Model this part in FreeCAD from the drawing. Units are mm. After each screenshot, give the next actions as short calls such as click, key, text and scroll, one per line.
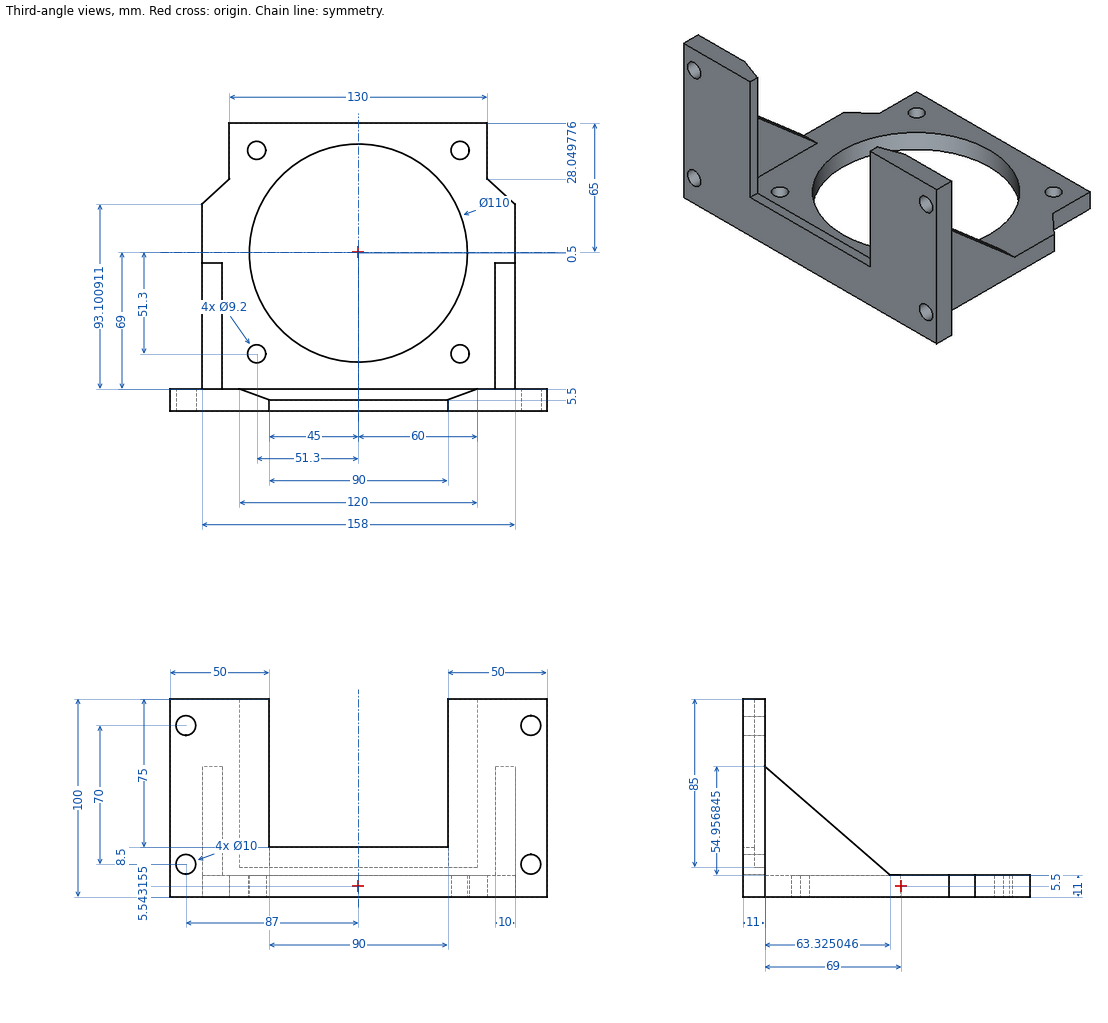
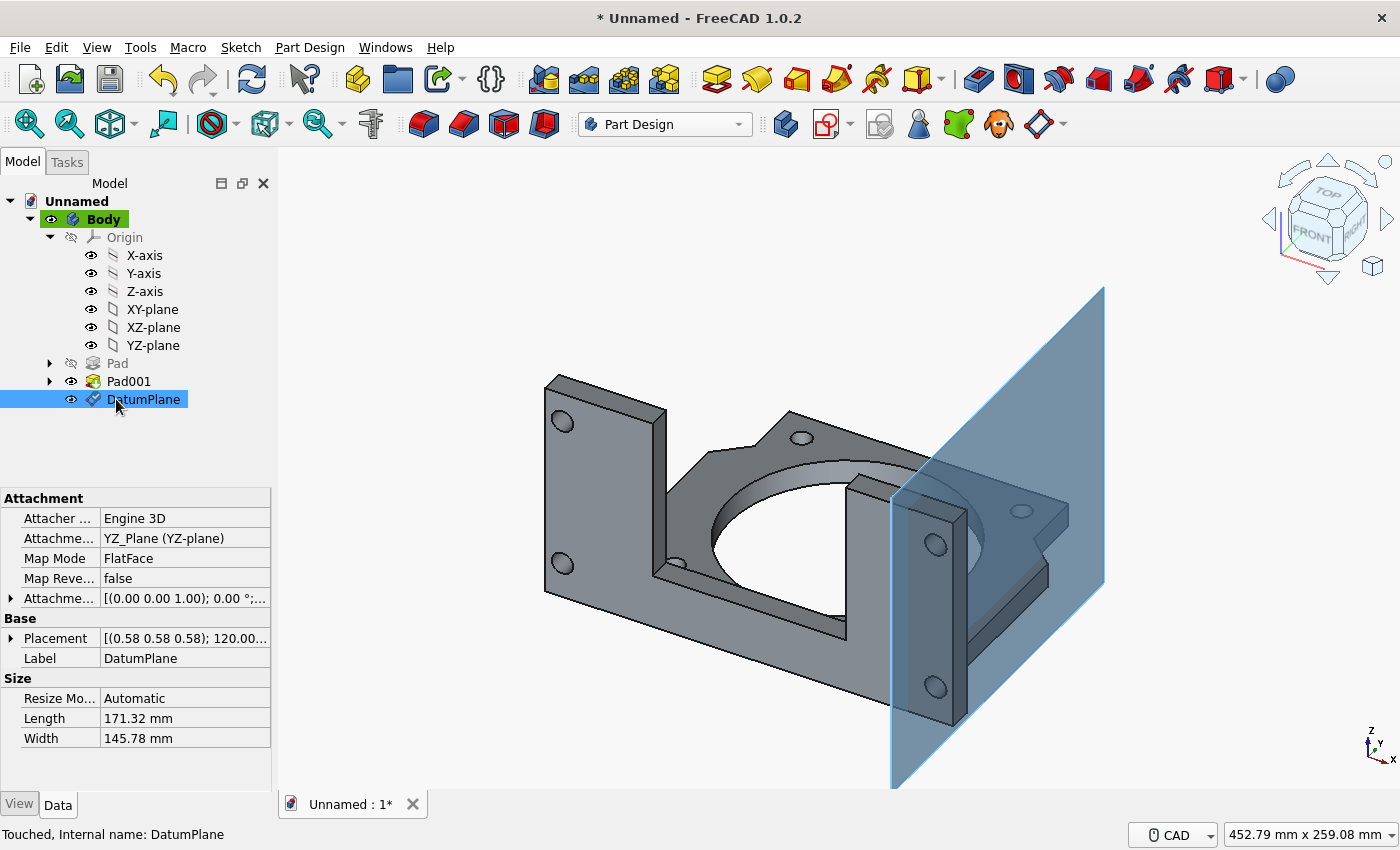
click(826, 124)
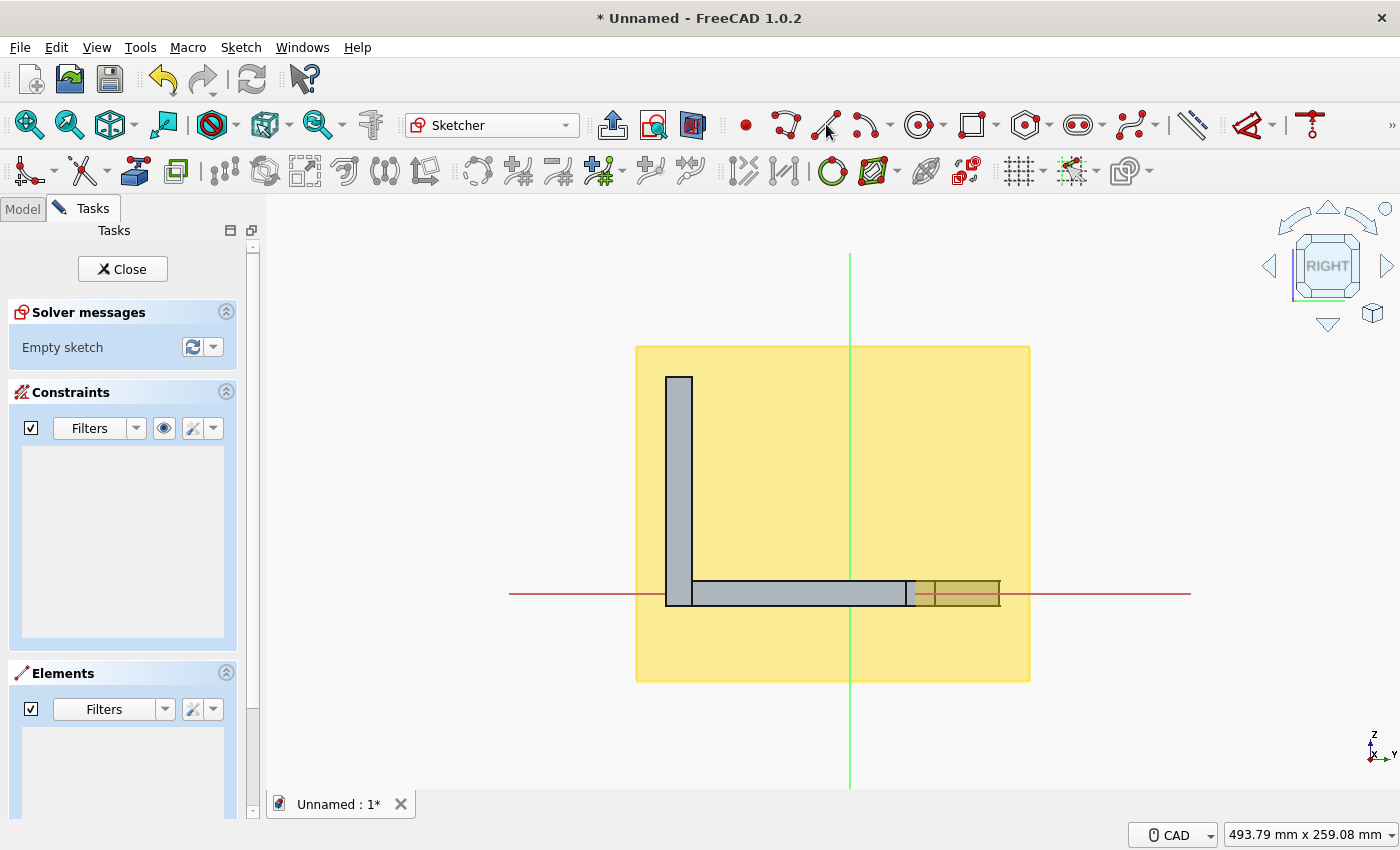
key(q)
key(s)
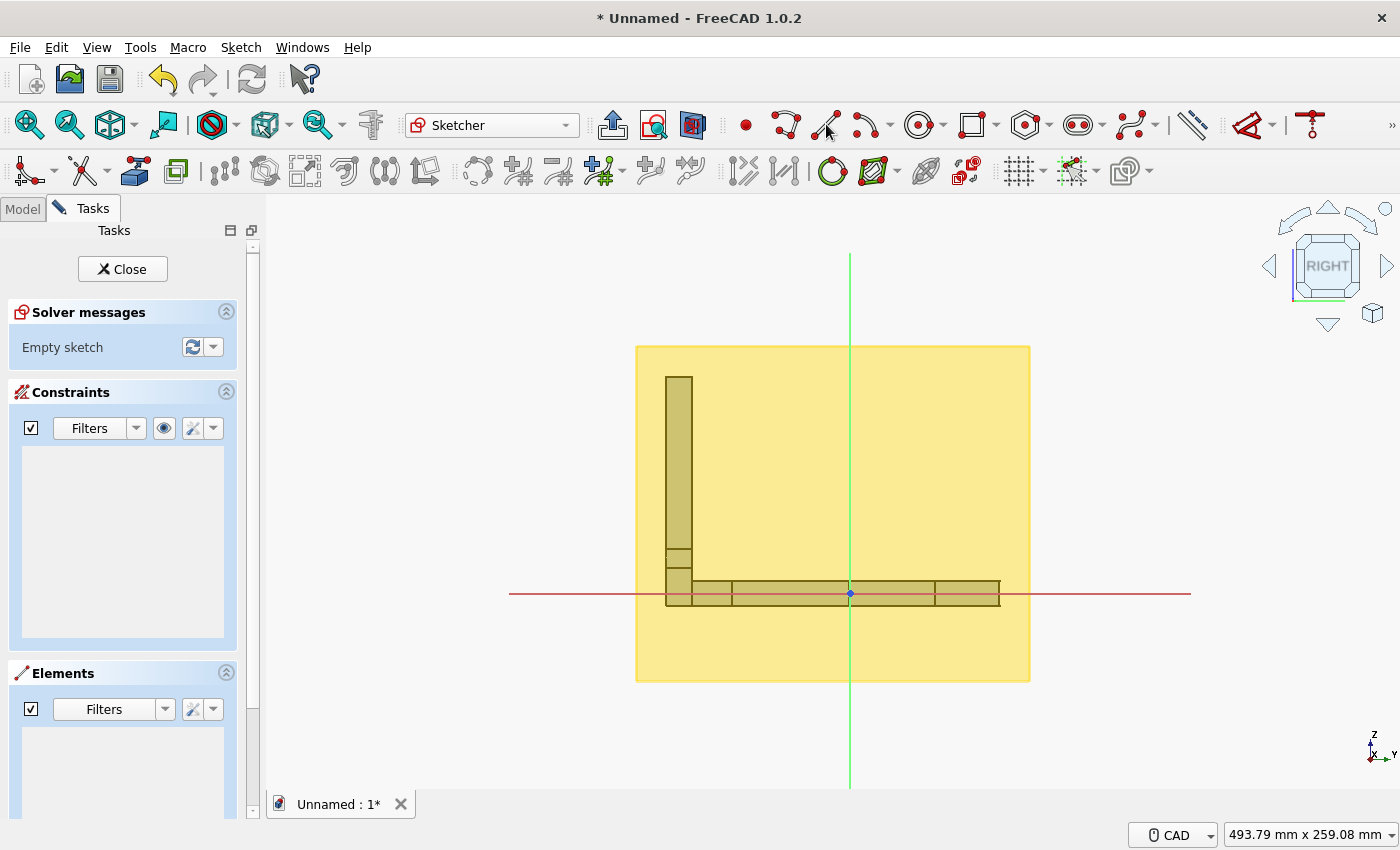
scroll(775, 543, up, 5)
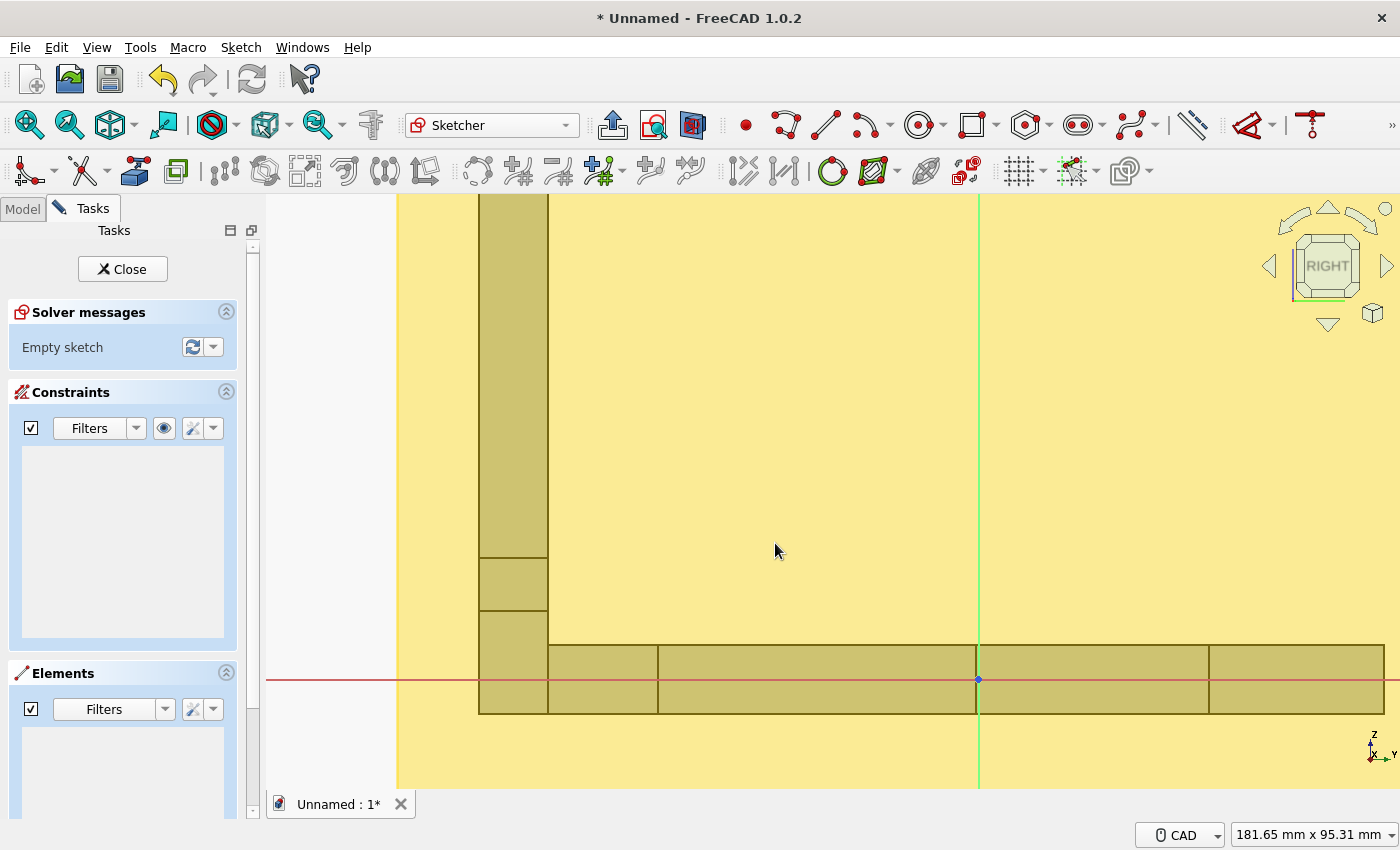
click(786, 126)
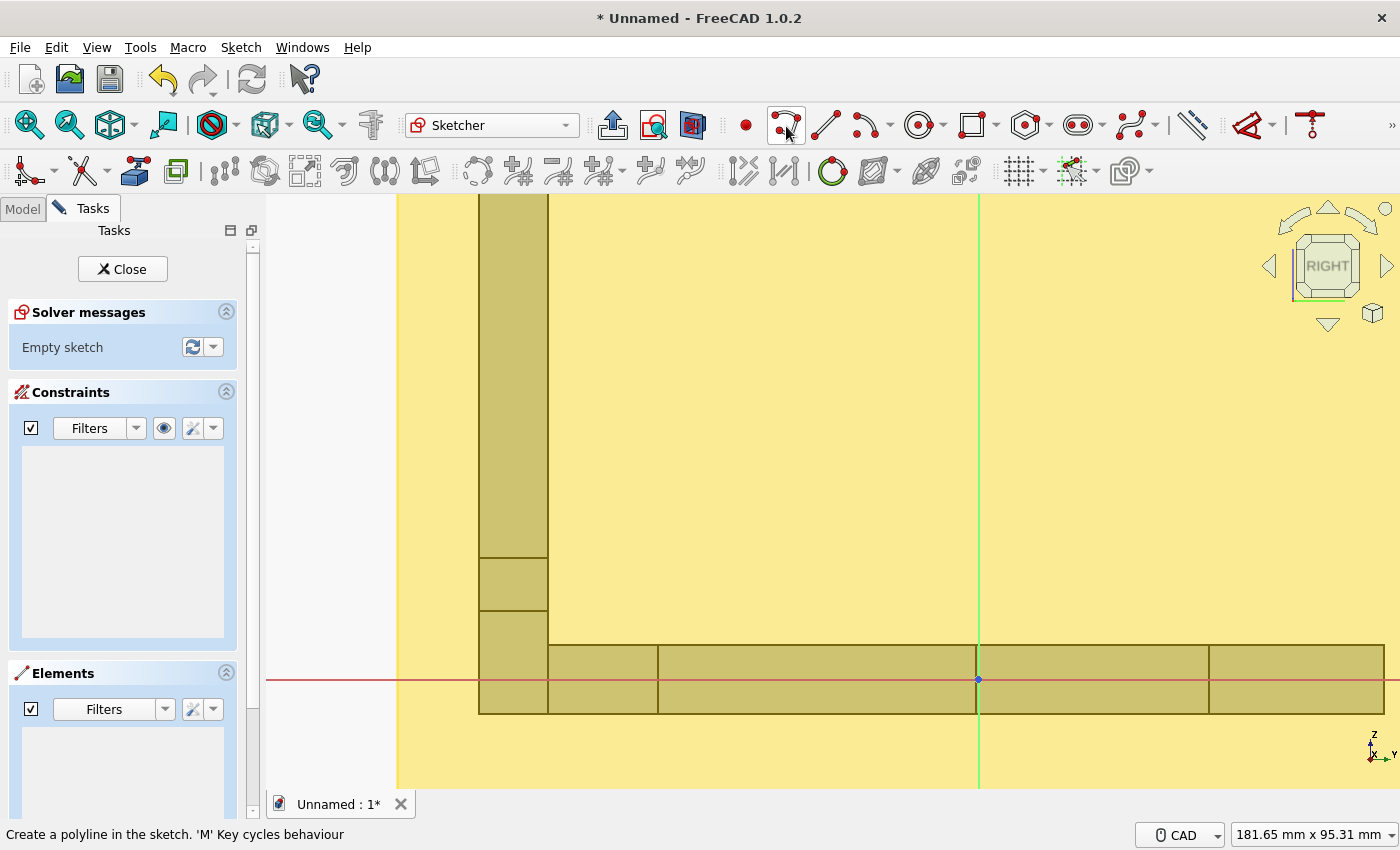
click(943, 645)
click(548, 302)
click(548, 645)
click(943, 646)
key(Escape)
key(Escape)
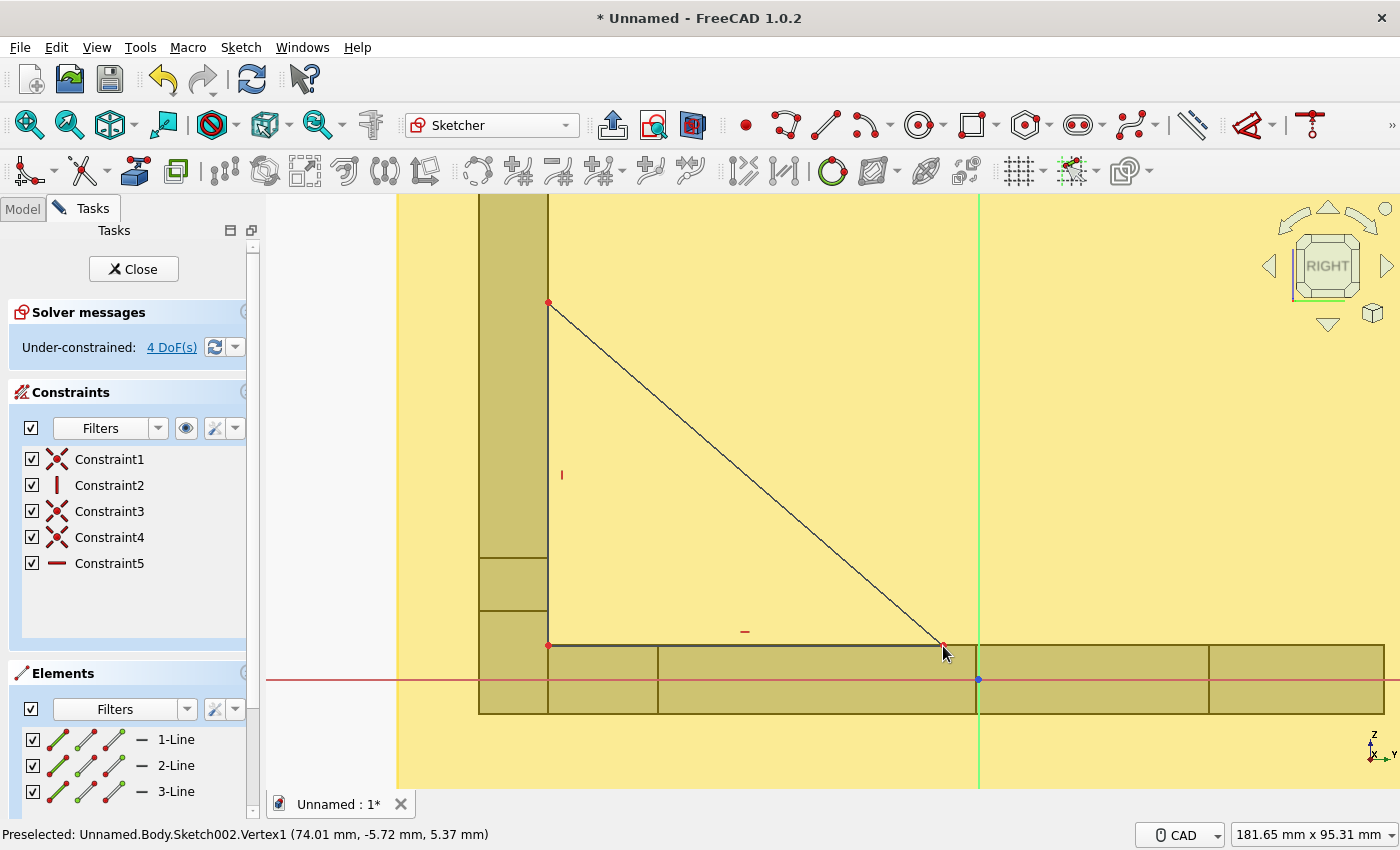
key(d)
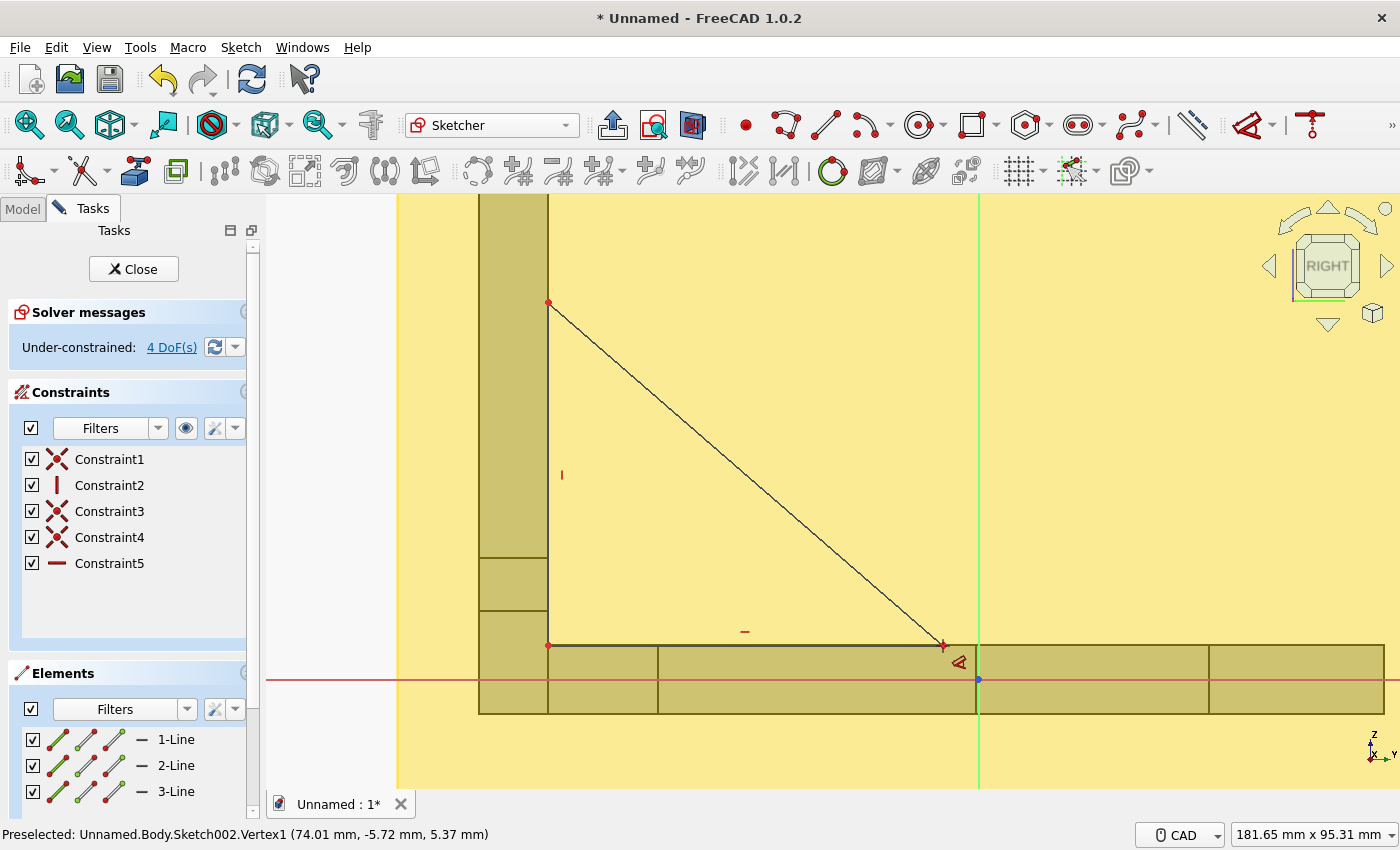
click(548, 303)
click(763, 714)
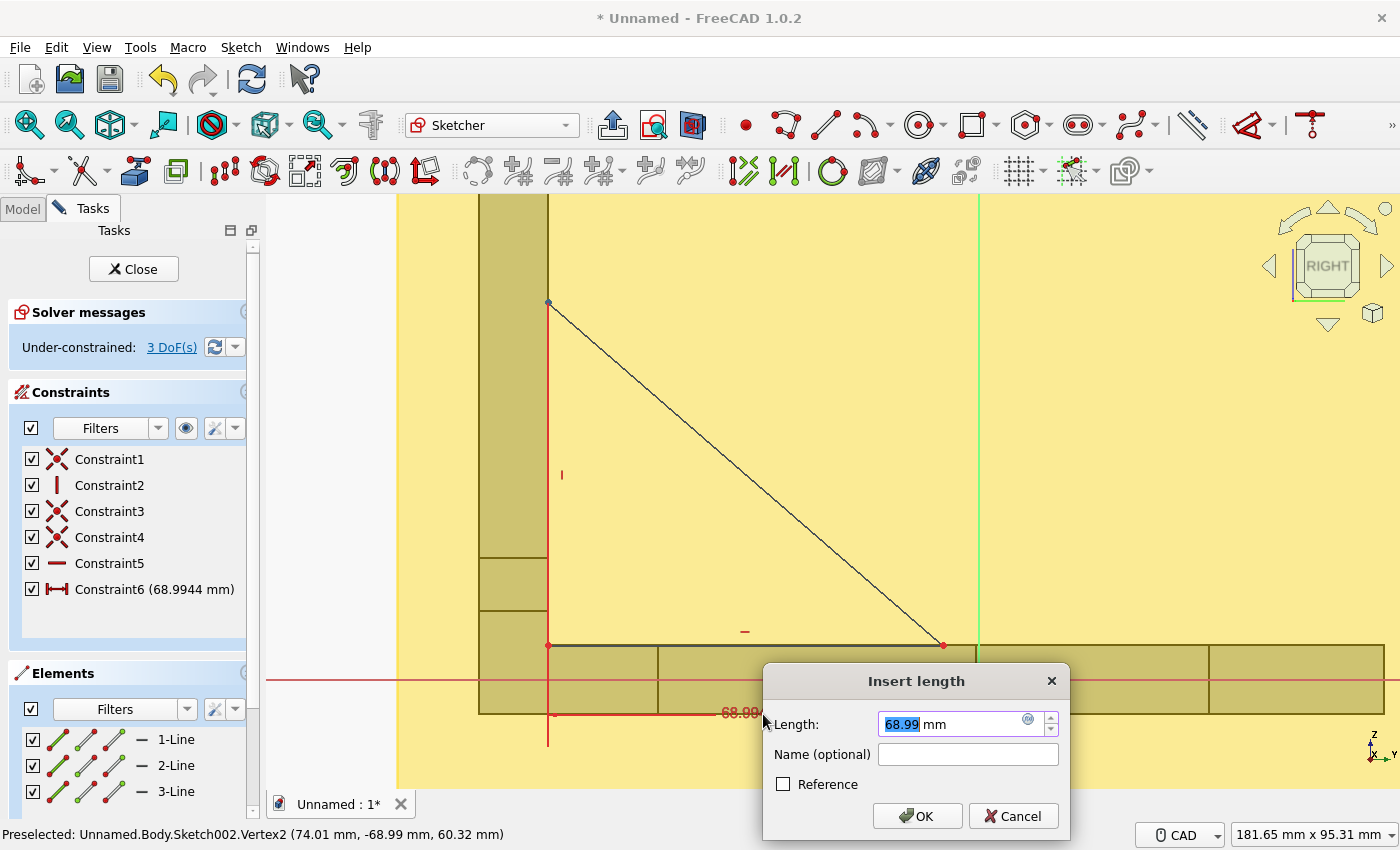
text(69)
key(Return)